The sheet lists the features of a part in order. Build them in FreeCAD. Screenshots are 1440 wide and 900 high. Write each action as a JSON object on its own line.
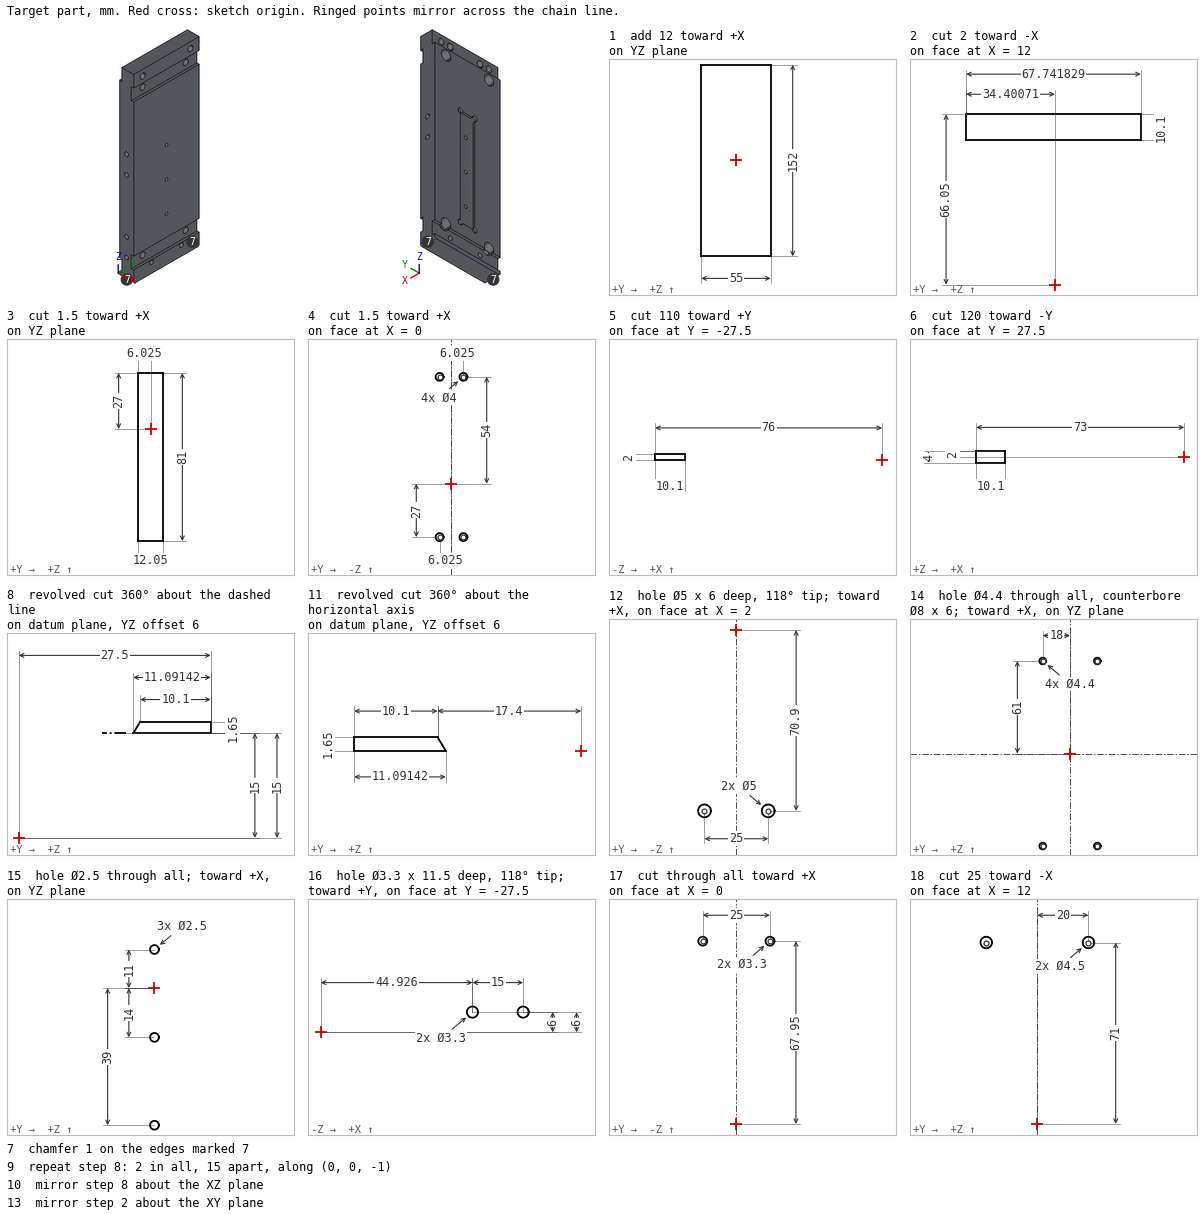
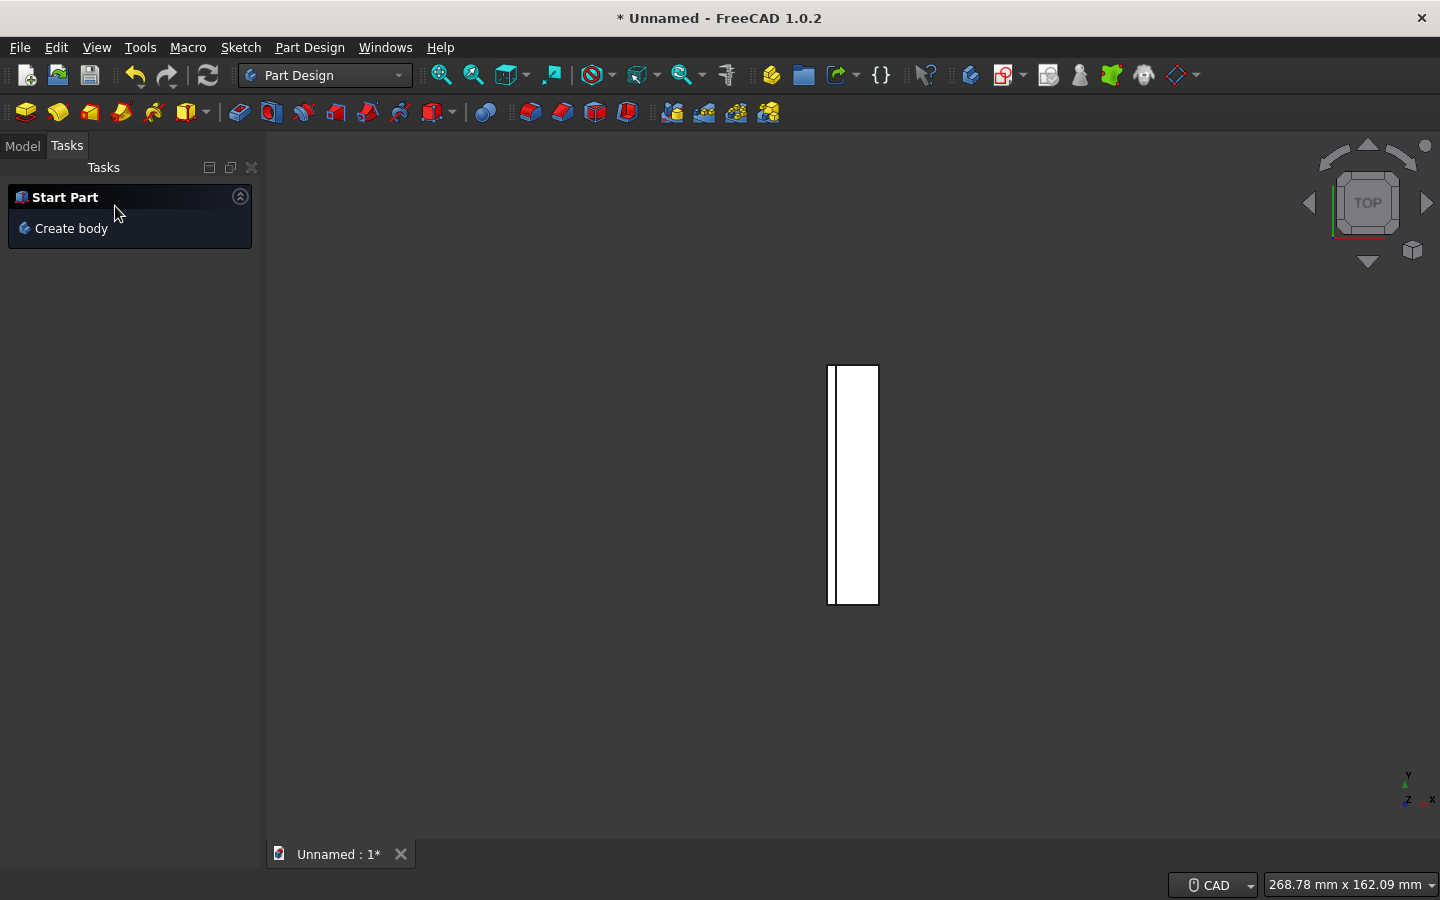
{"action": "key", "text": "1"}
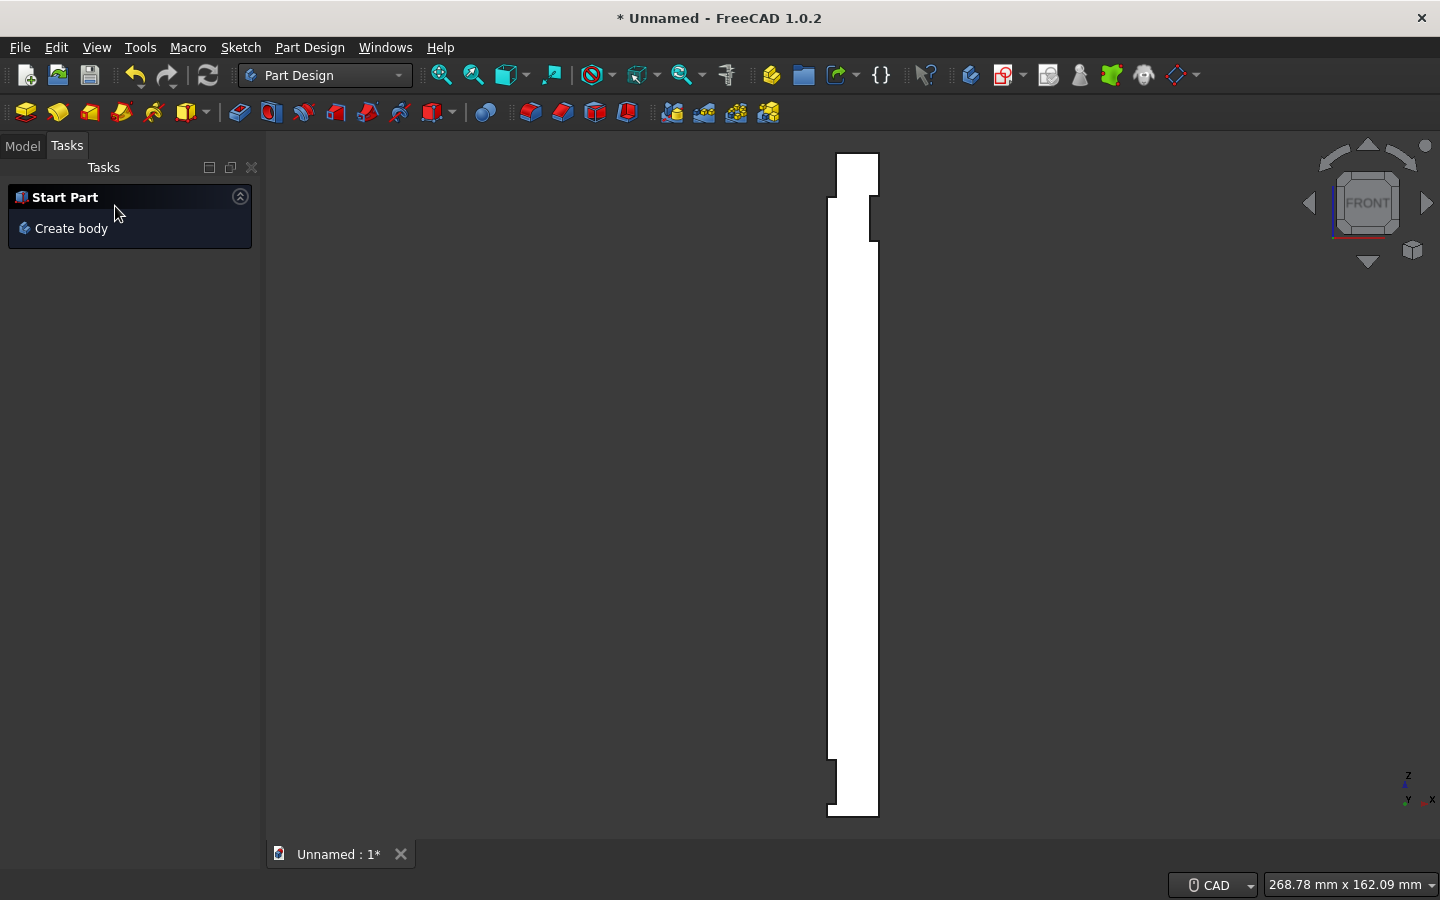
{"action": "key", "text": "3"}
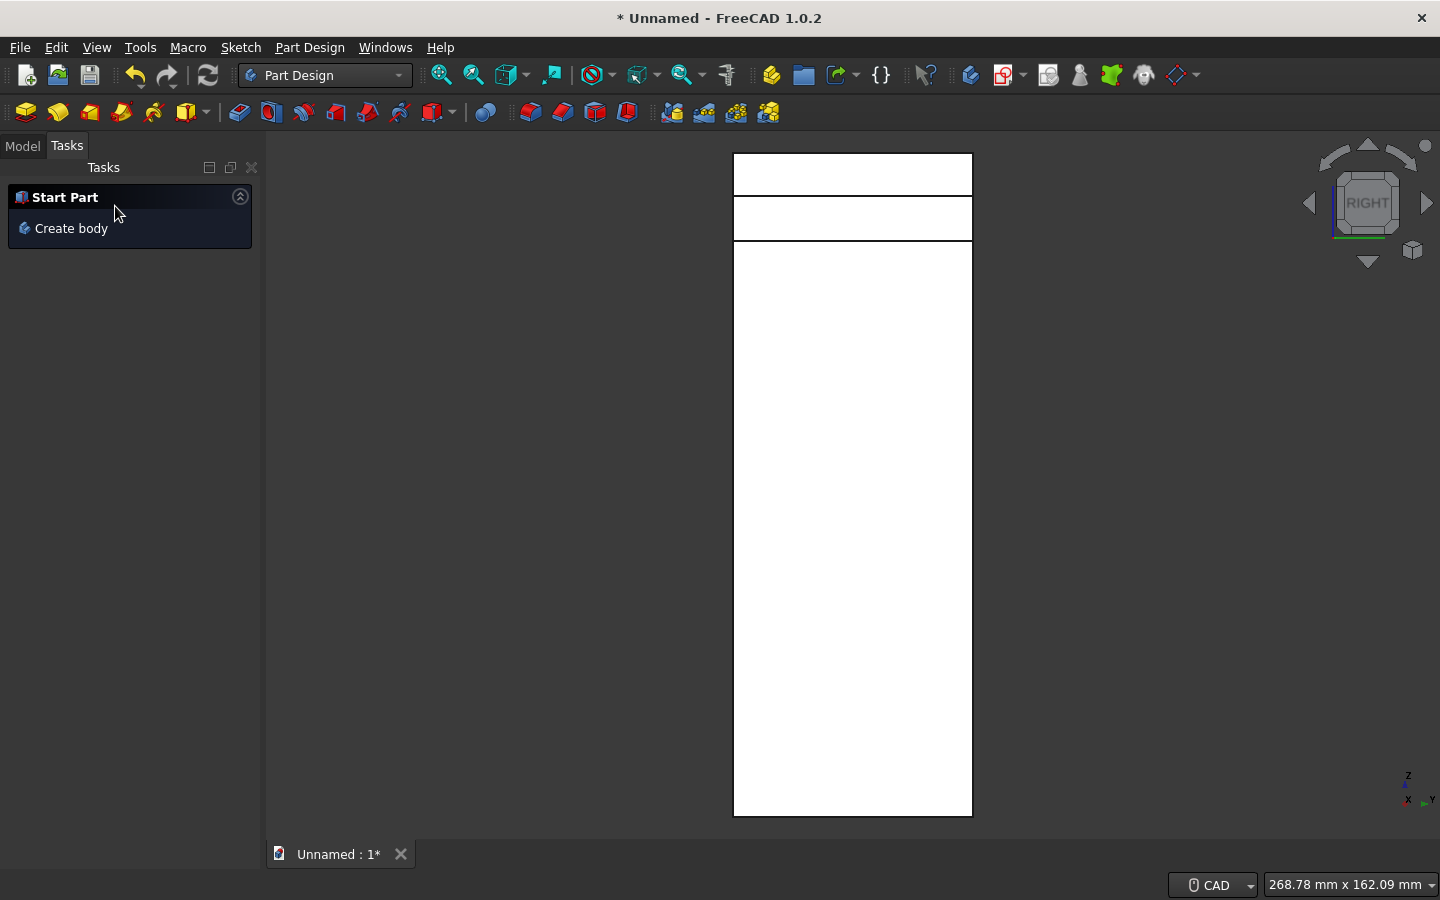
{"action": "key", "text": "5"}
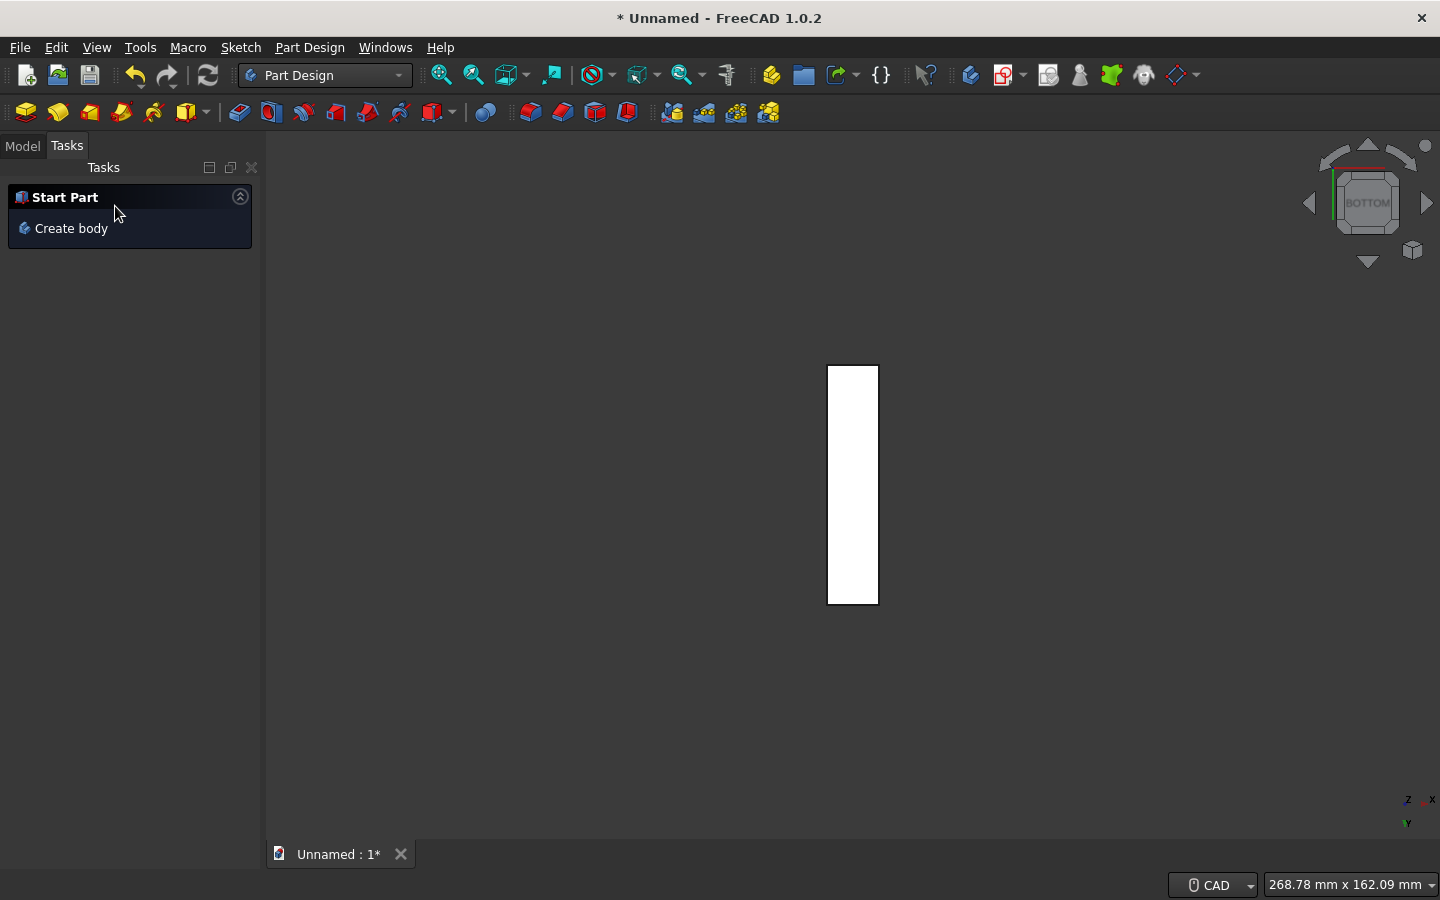
{"action": "left_click", "coordinate": [442, 76]}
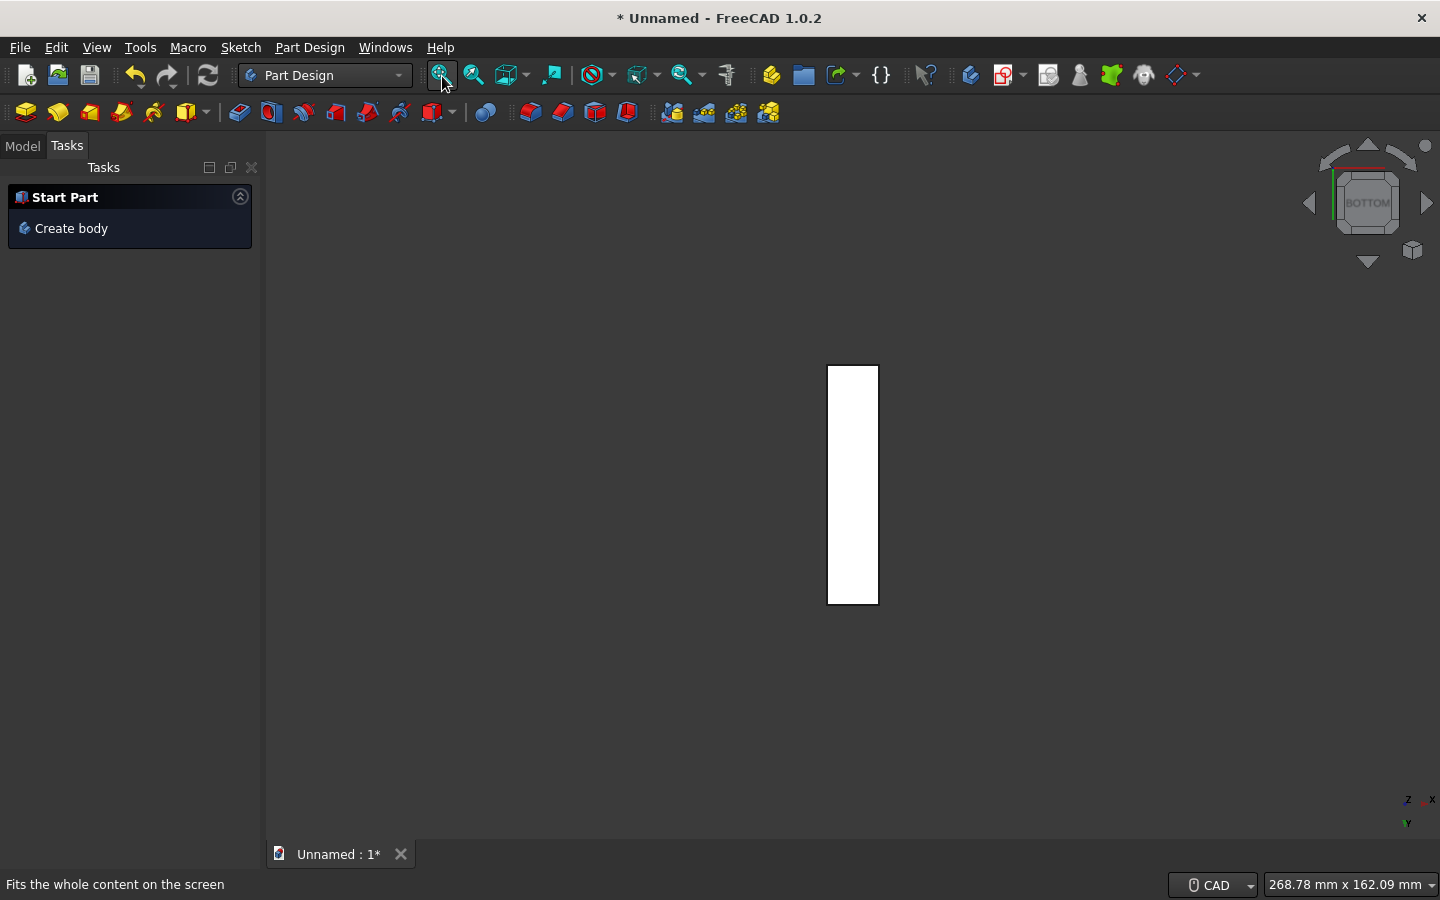
{"action": "left_click", "coordinate": [853, 364]}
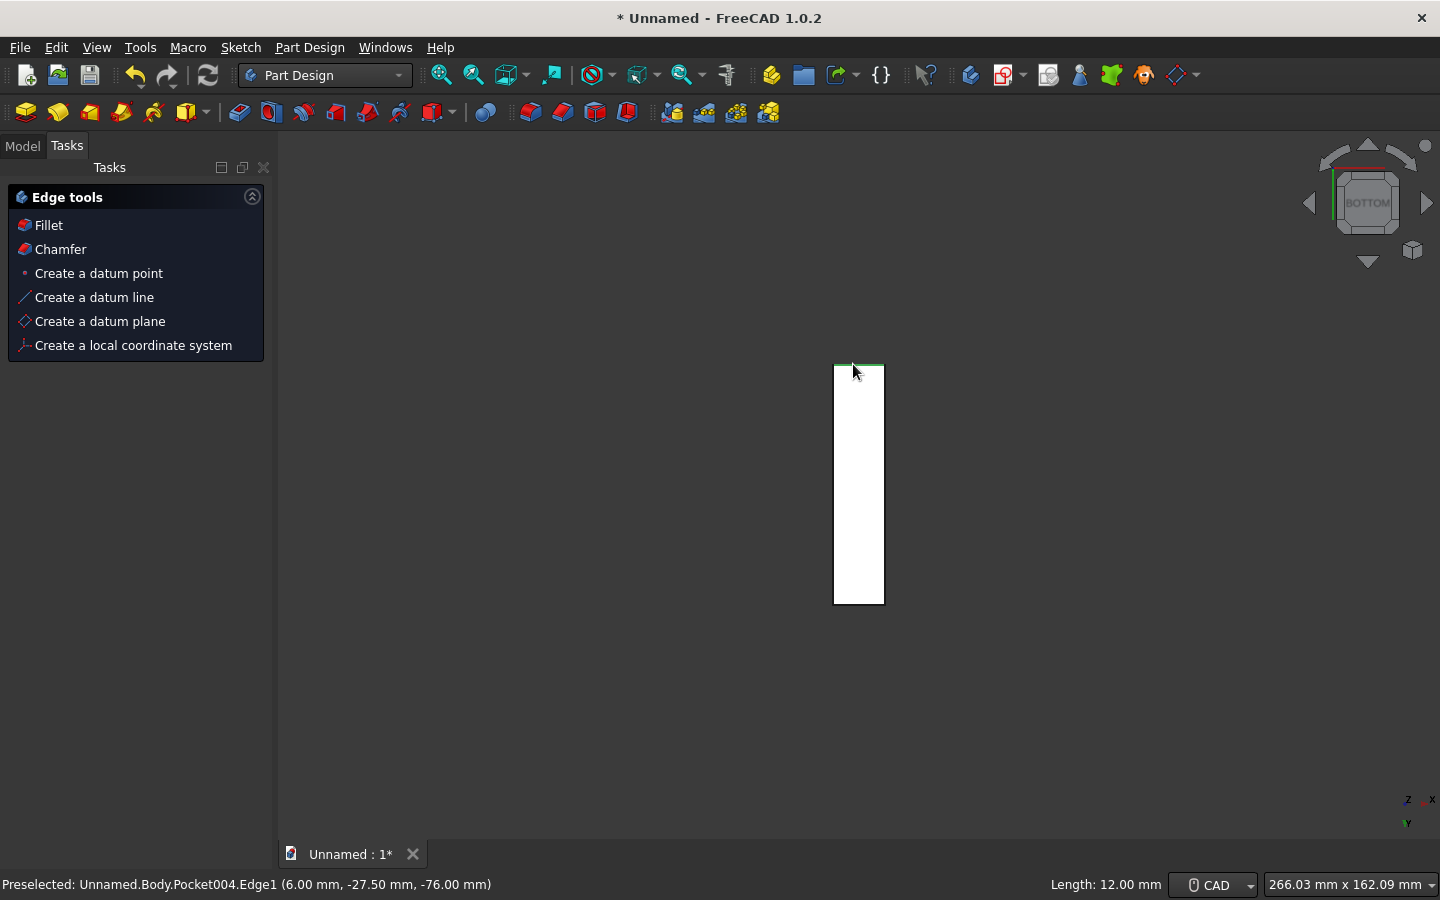
{"action": "left_click", "coordinate": [859, 604], "text": "ctrl"}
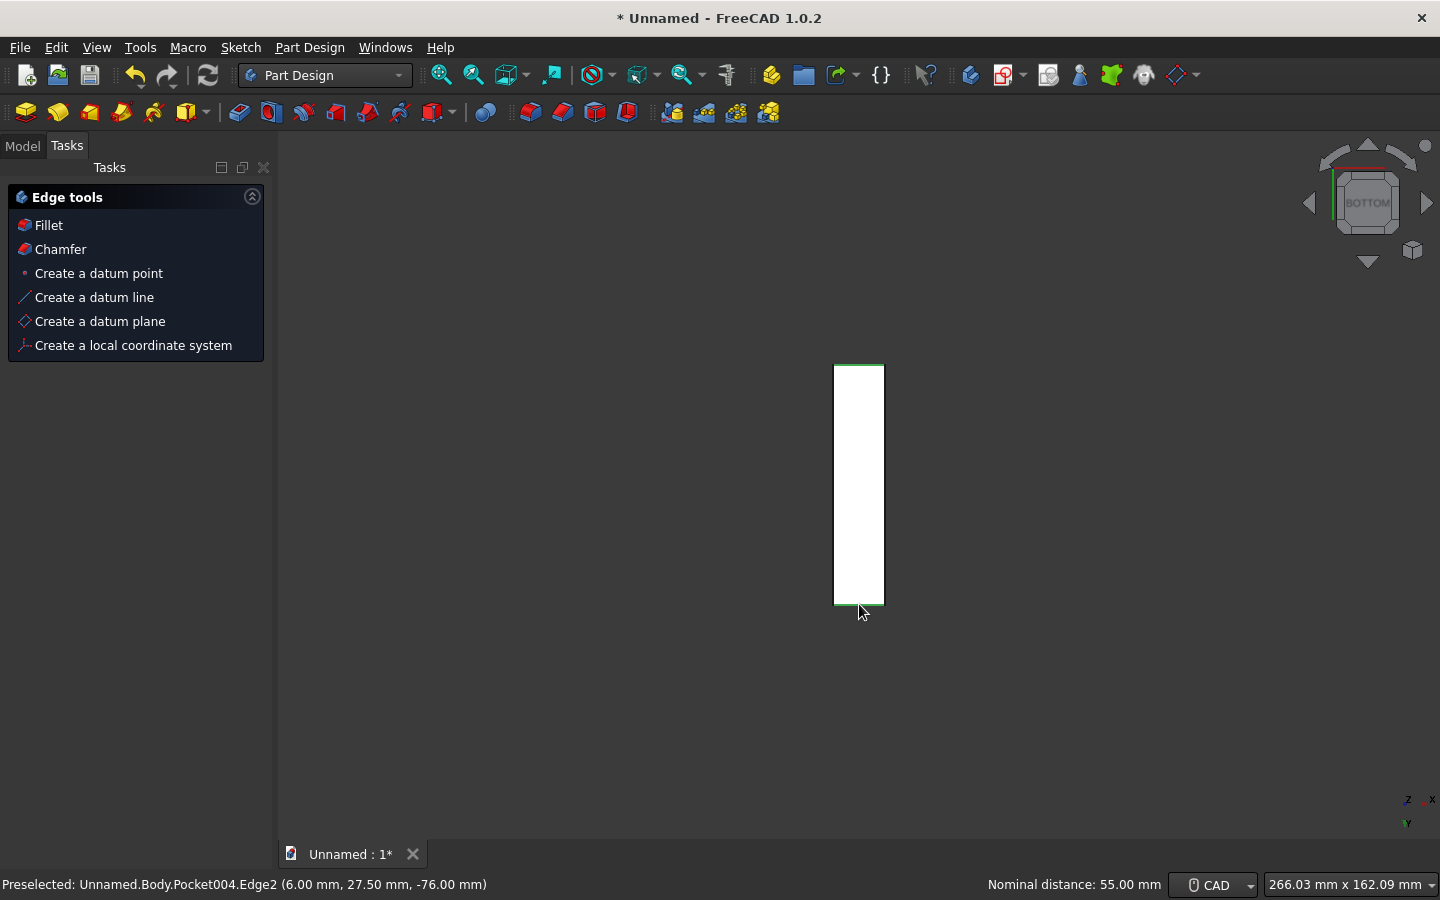
{"action": "left_click", "coordinate": [564, 112]}